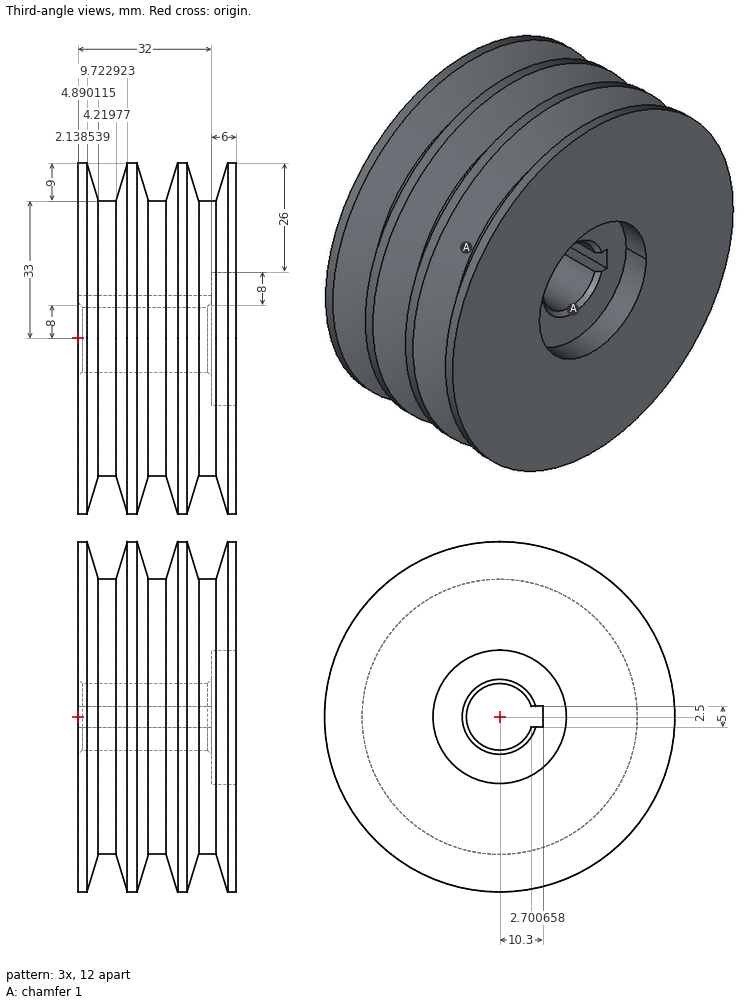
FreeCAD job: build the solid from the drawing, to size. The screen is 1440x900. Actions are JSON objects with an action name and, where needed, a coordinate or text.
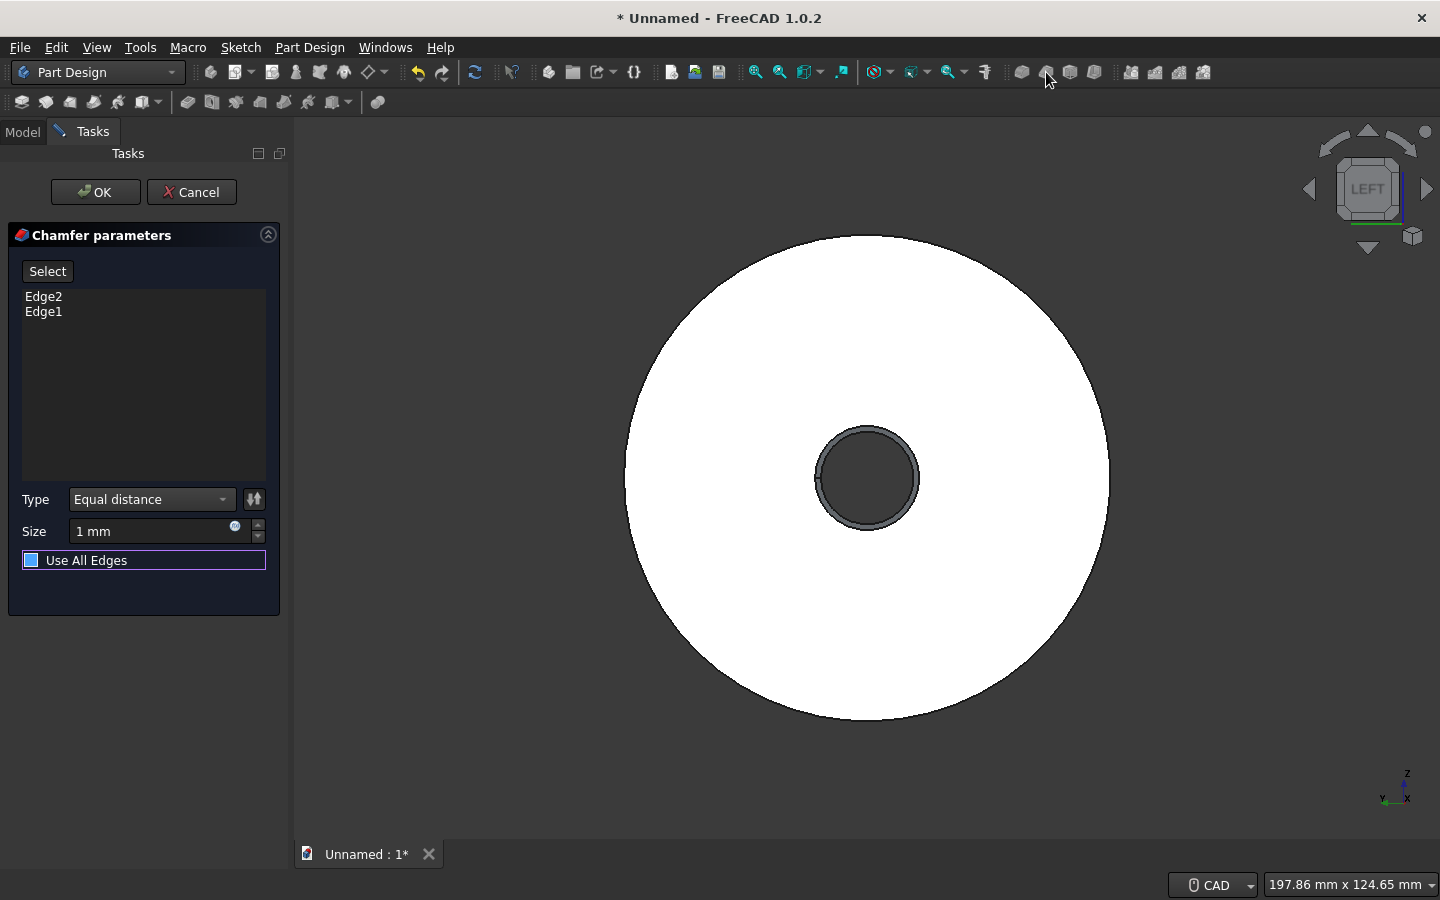
{"action": "left_click", "coordinate": [96, 192]}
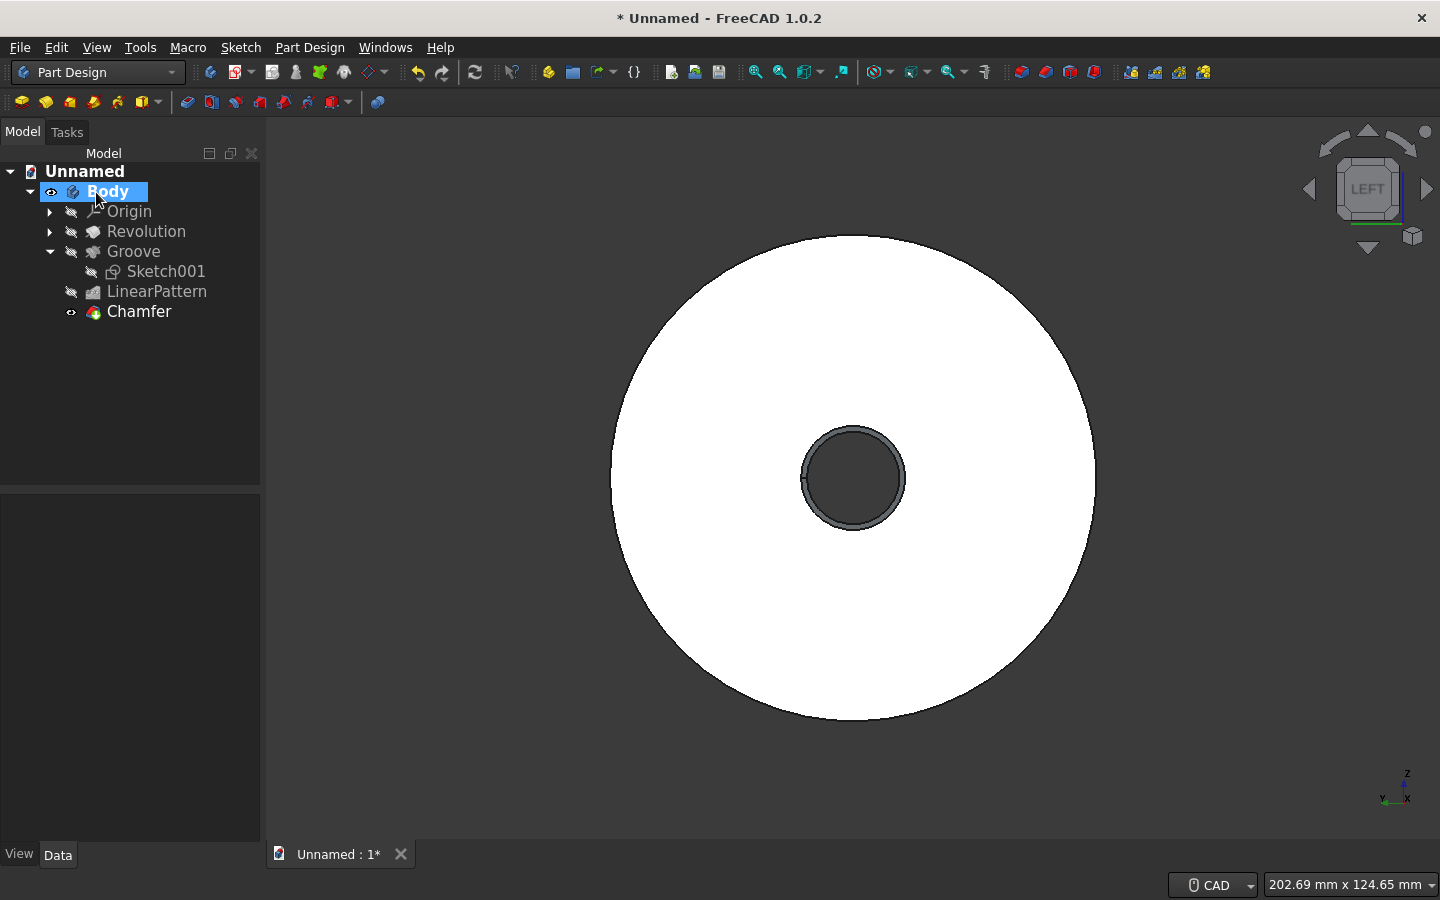
{"action": "left_click", "coordinate": [236, 72]}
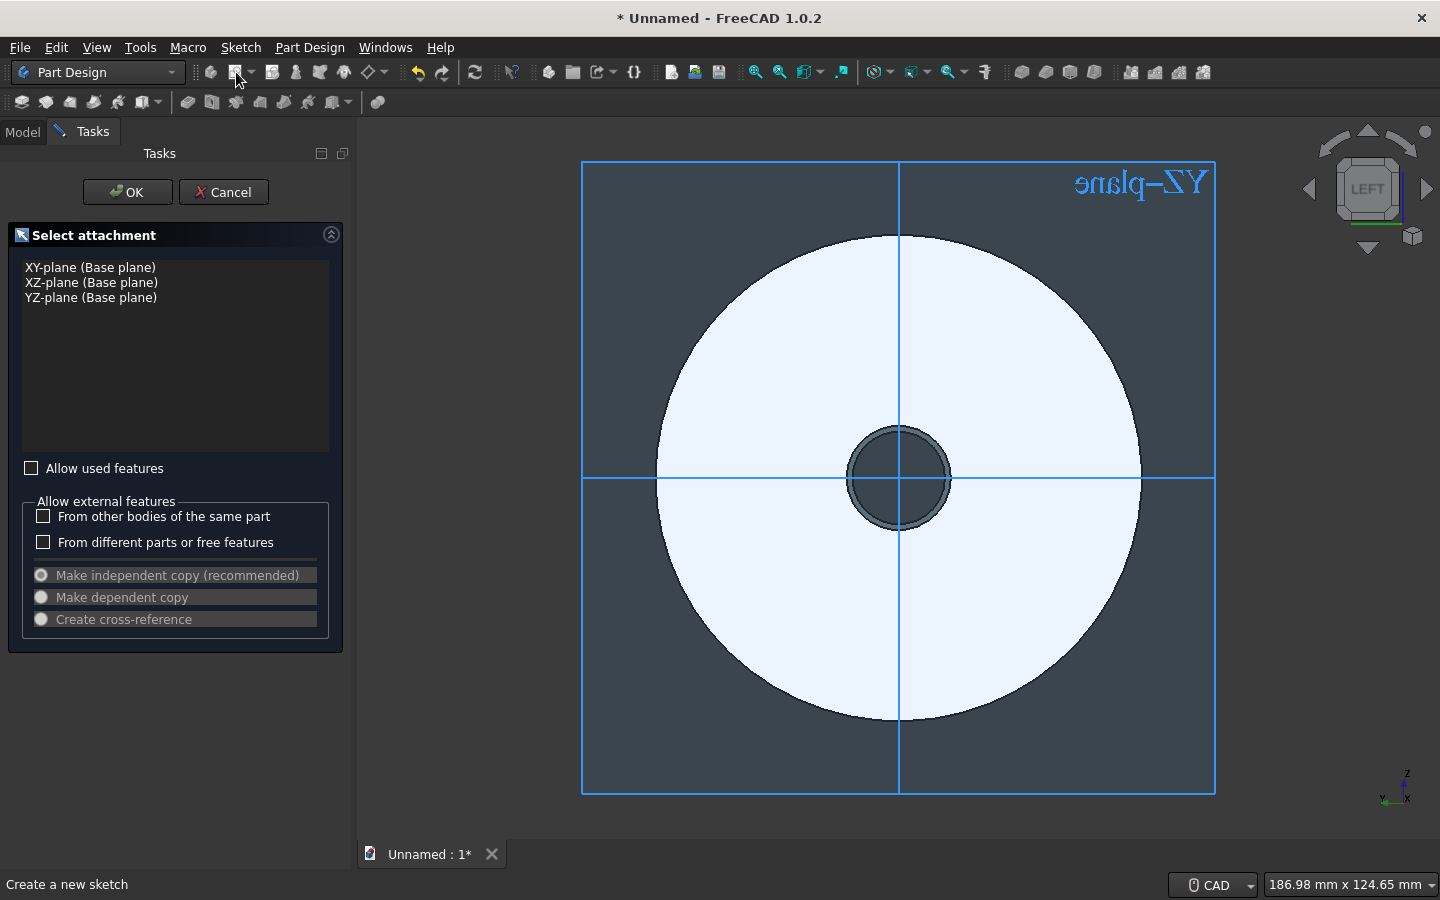
{"action": "left_click", "coordinate": [82, 298]}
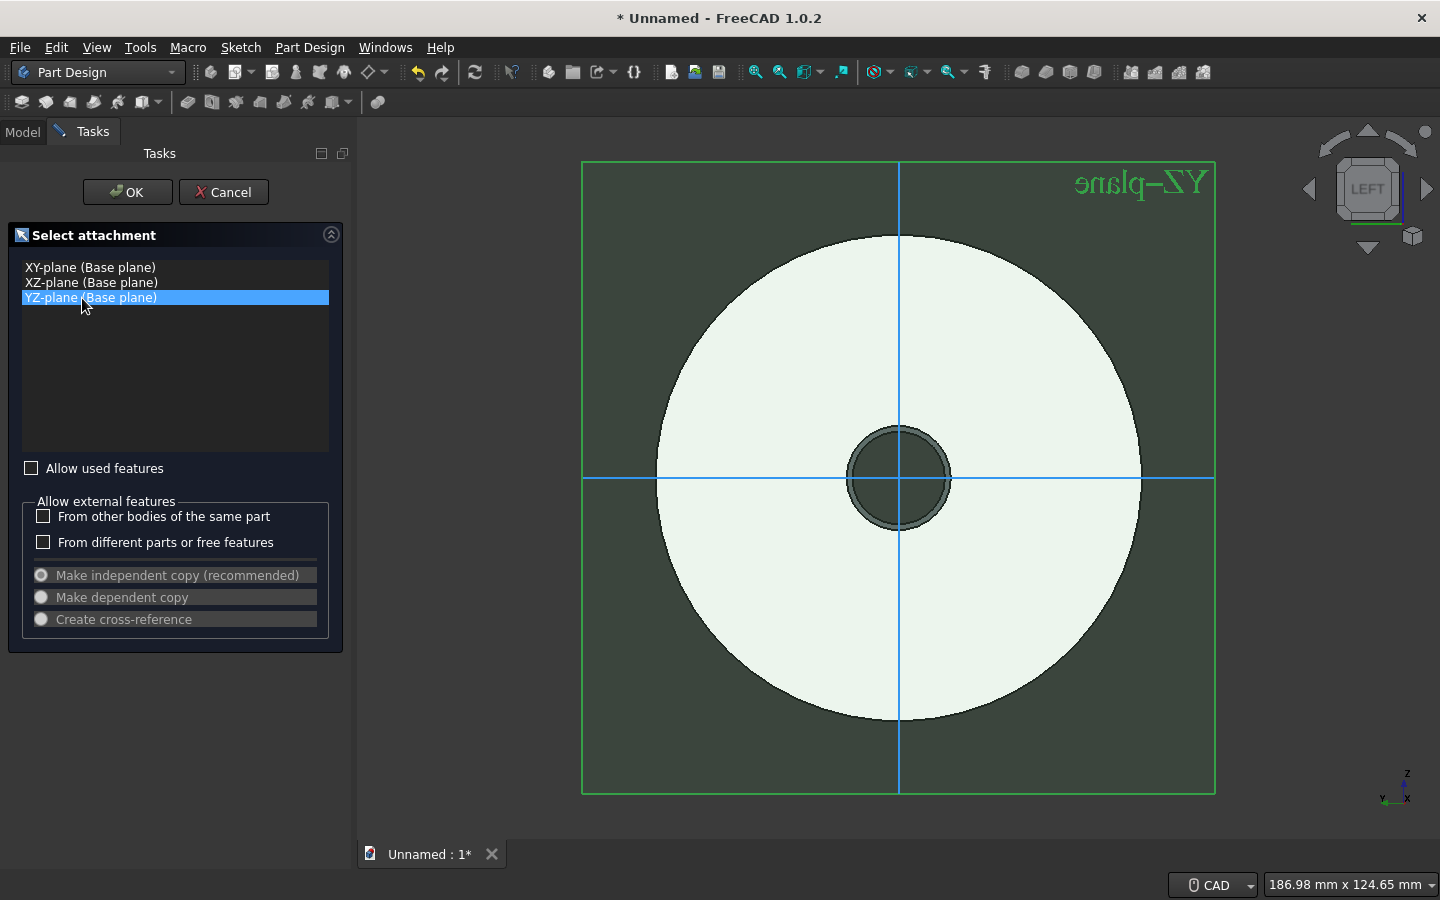
{"action": "left_click", "coordinate": [128, 192]}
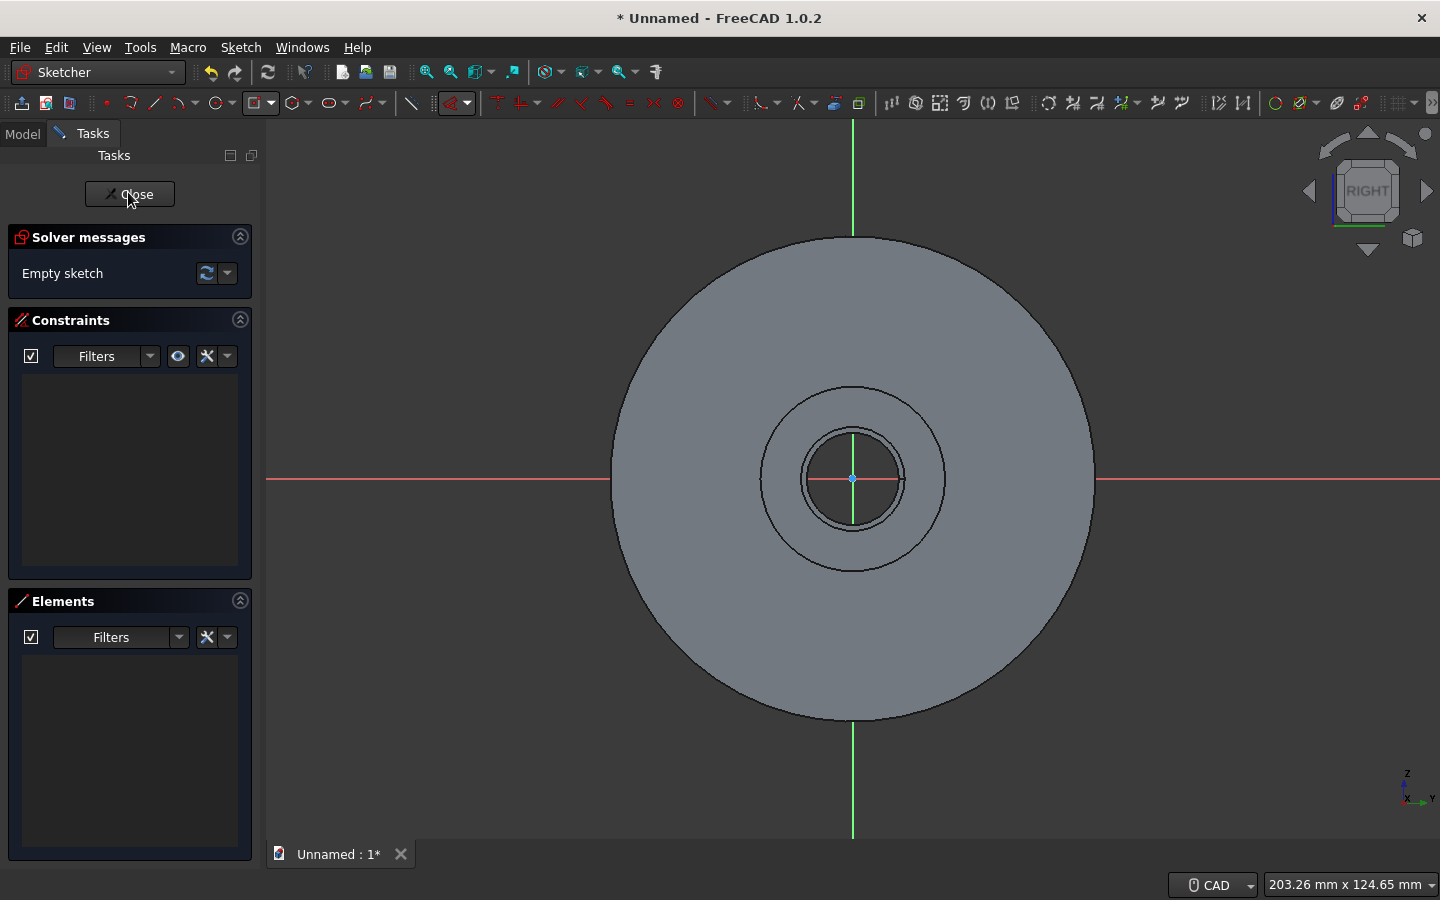
{"action": "key", "text": "q s"}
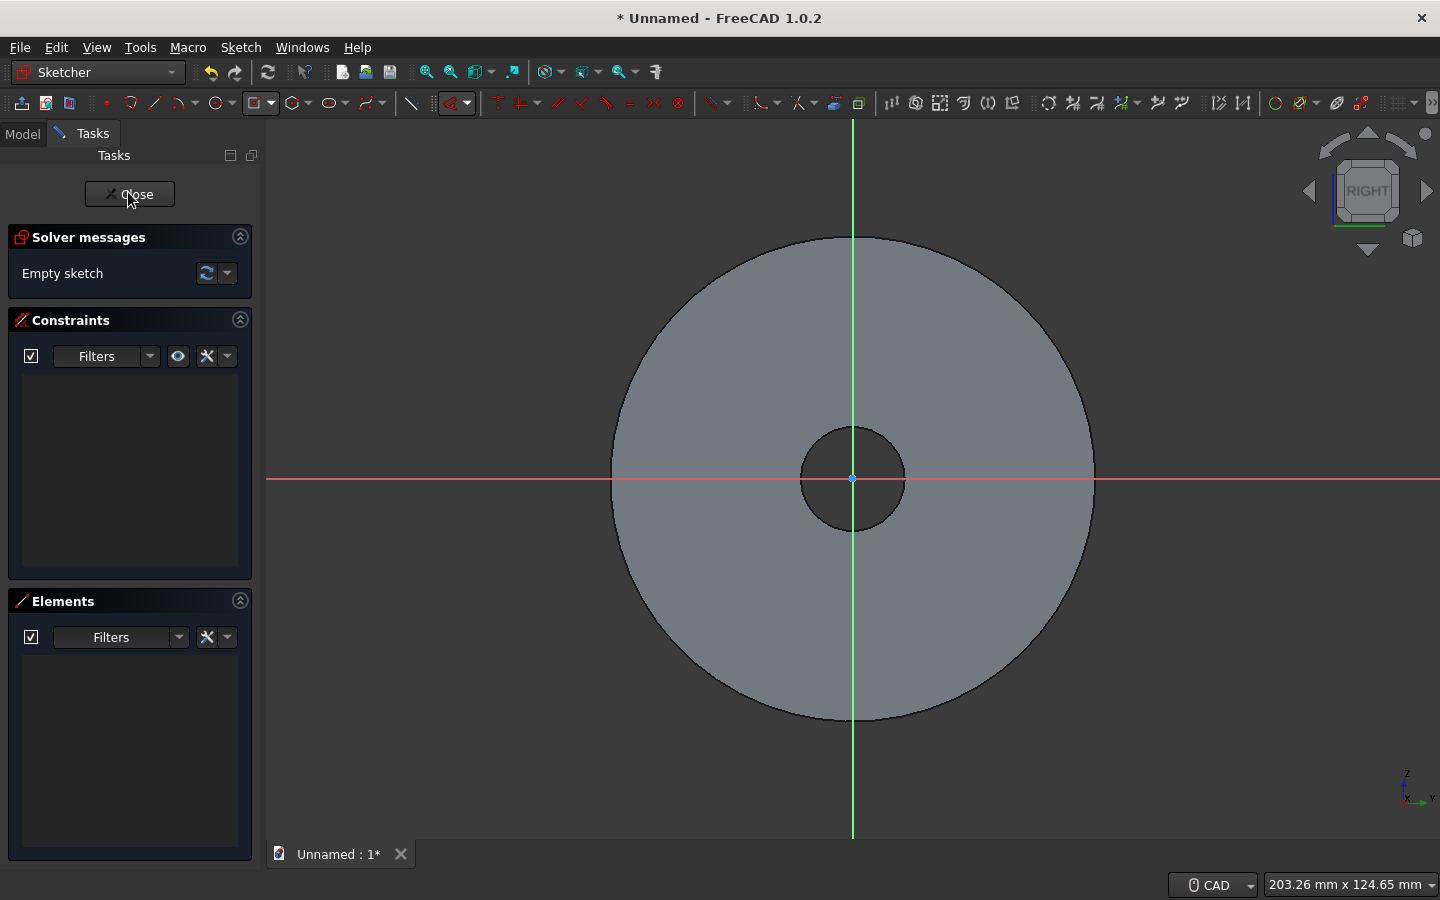
{"action": "scroll", "coordinate": [892, 479], "scroll_direction": "up", "scroll_amount": 12}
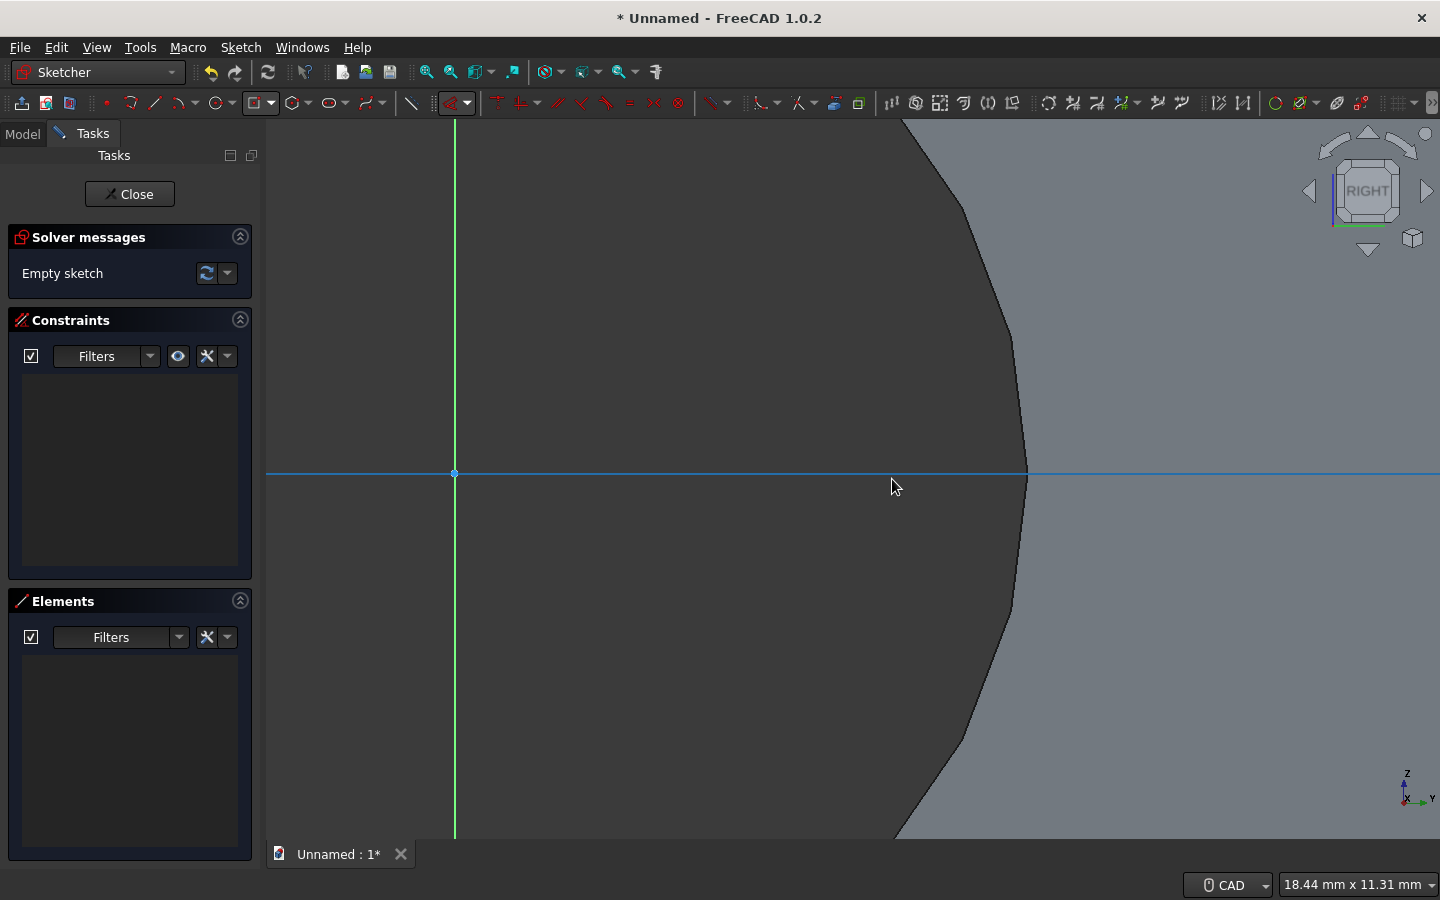
{"action": "key", "text": "g r"}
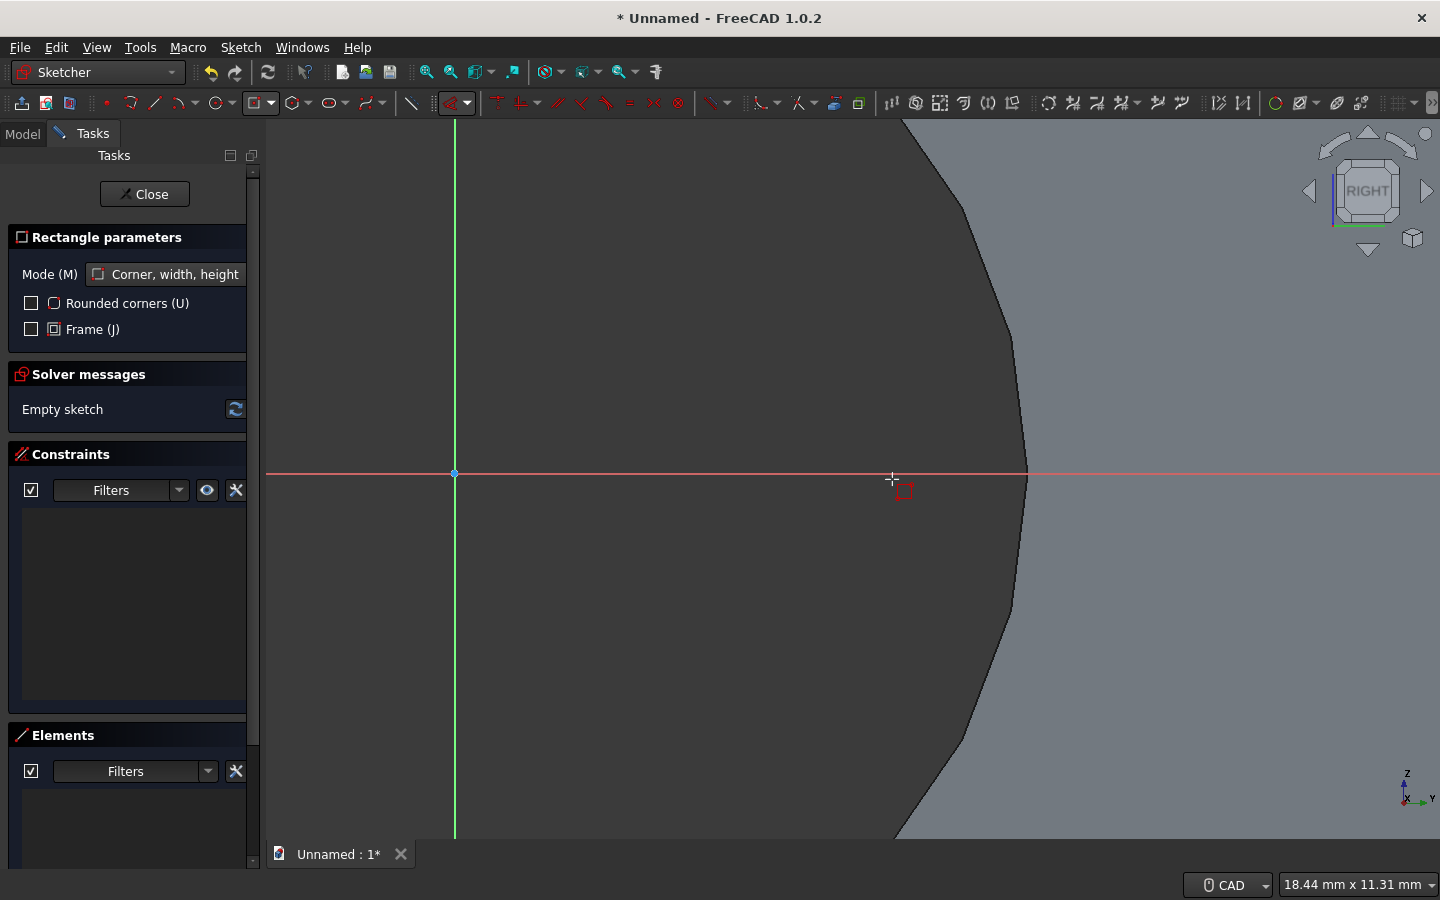
{"action": "left_click", "coordinate": [938, 315]}
{"action": "left_click", "coordinate": [1110, 633]}
{"action": "key", "text": "Escape"}